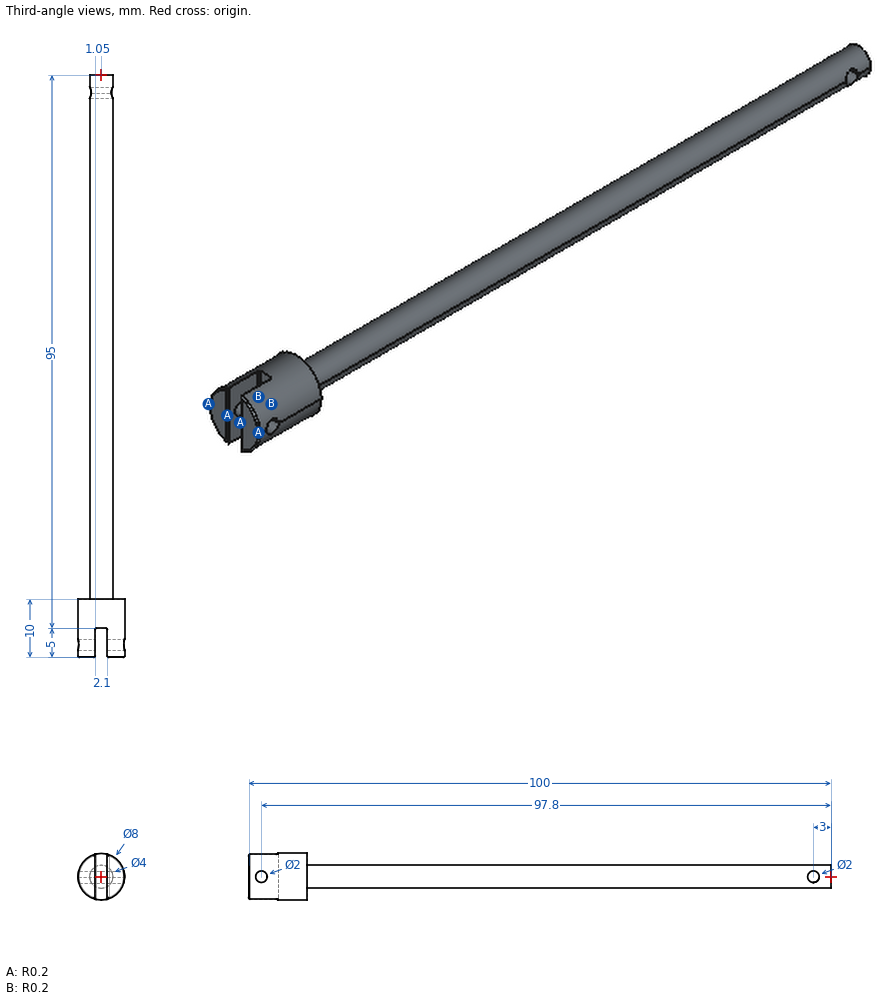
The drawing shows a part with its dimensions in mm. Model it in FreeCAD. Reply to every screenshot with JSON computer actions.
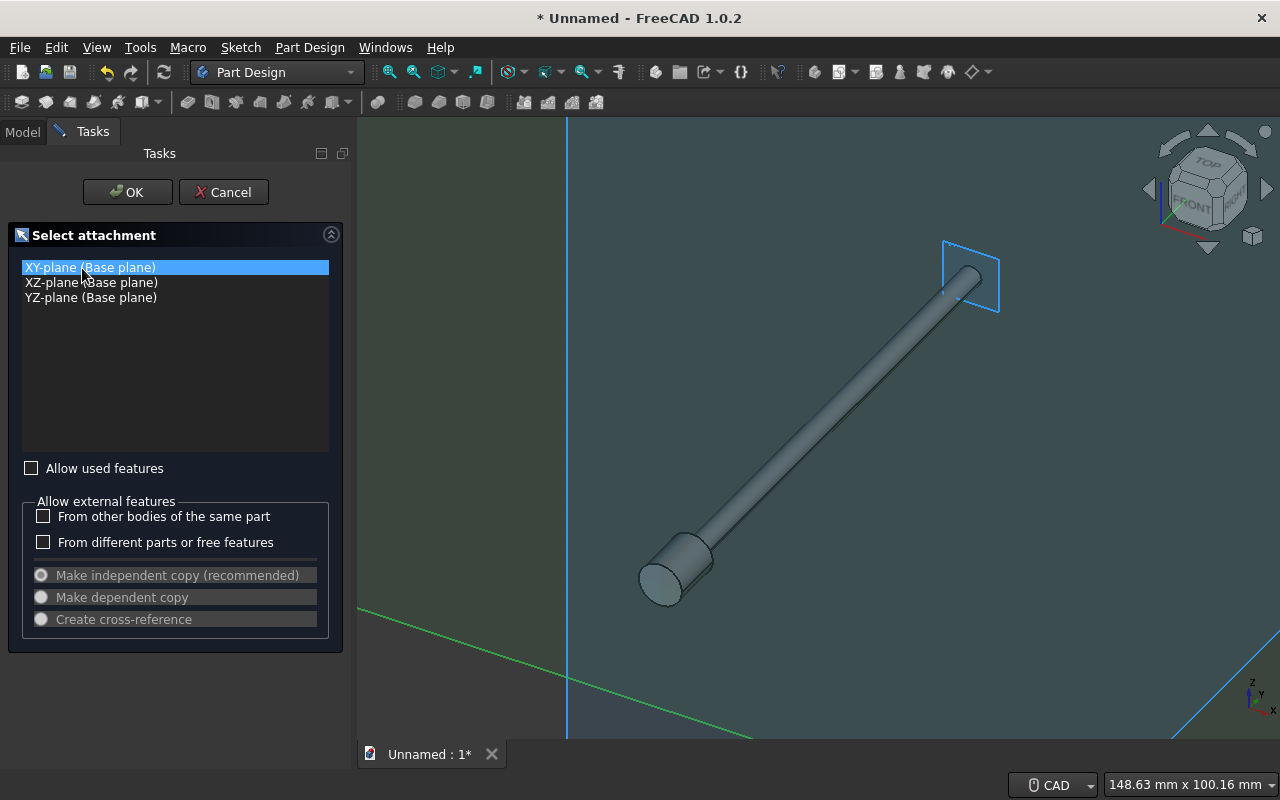
{"action": "left_click", "coordinate": [128, 192]}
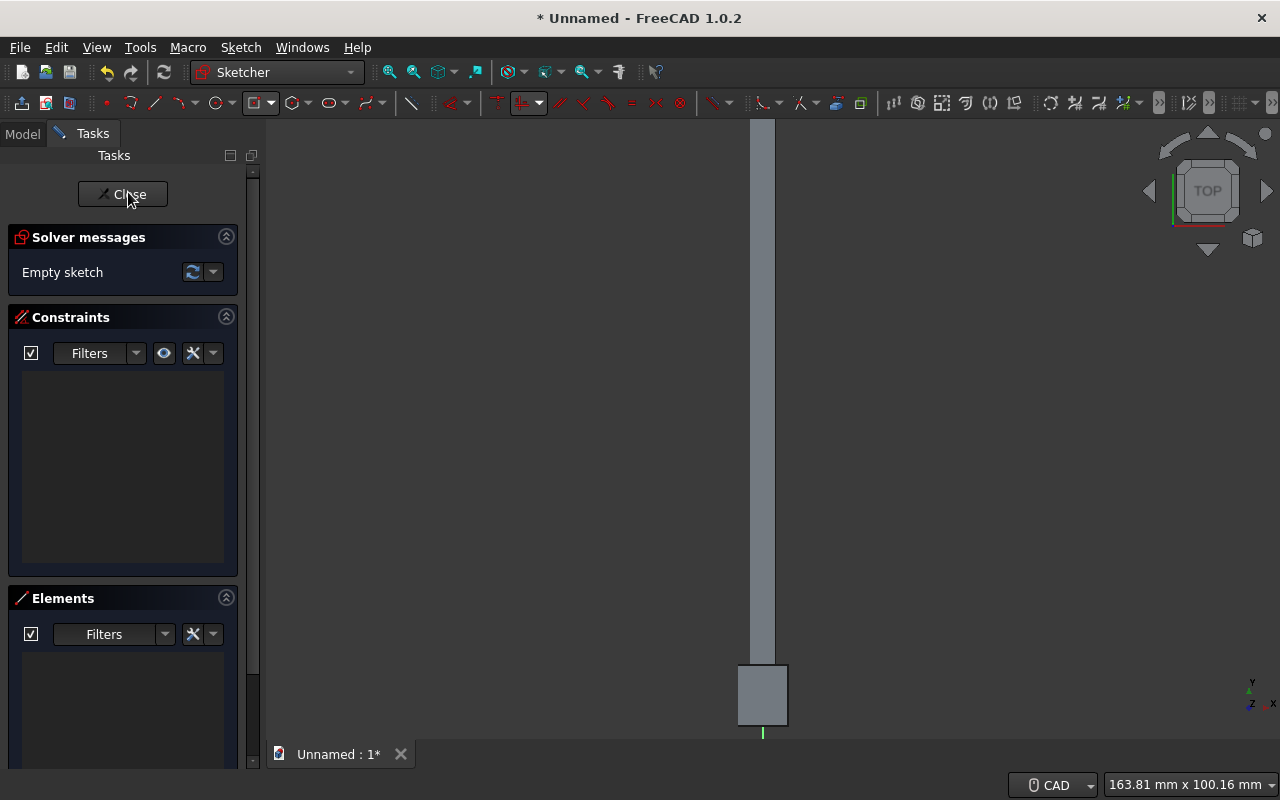
{"action": "key", "text": "q s"}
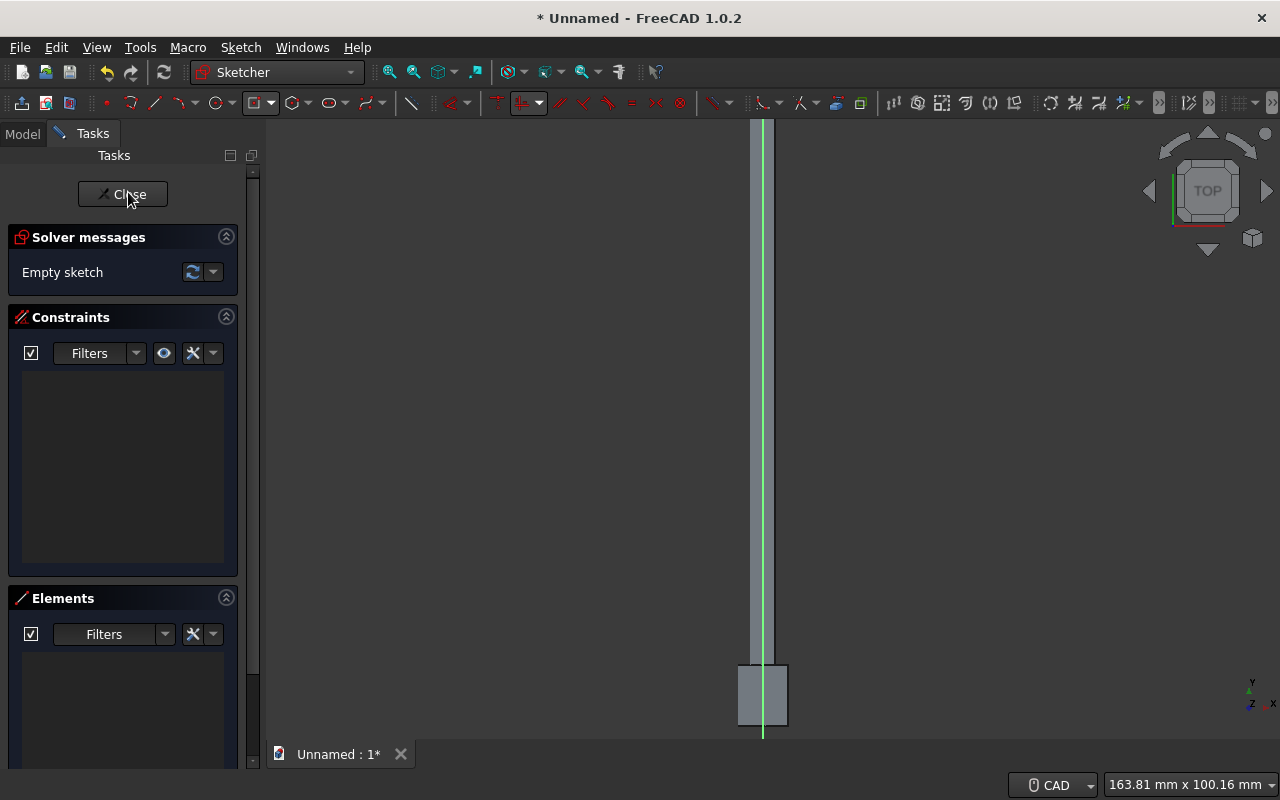
{"action": "scroll", "coordinate": [704, 429], "scroll_direction": "down", "scroll_amount": 5}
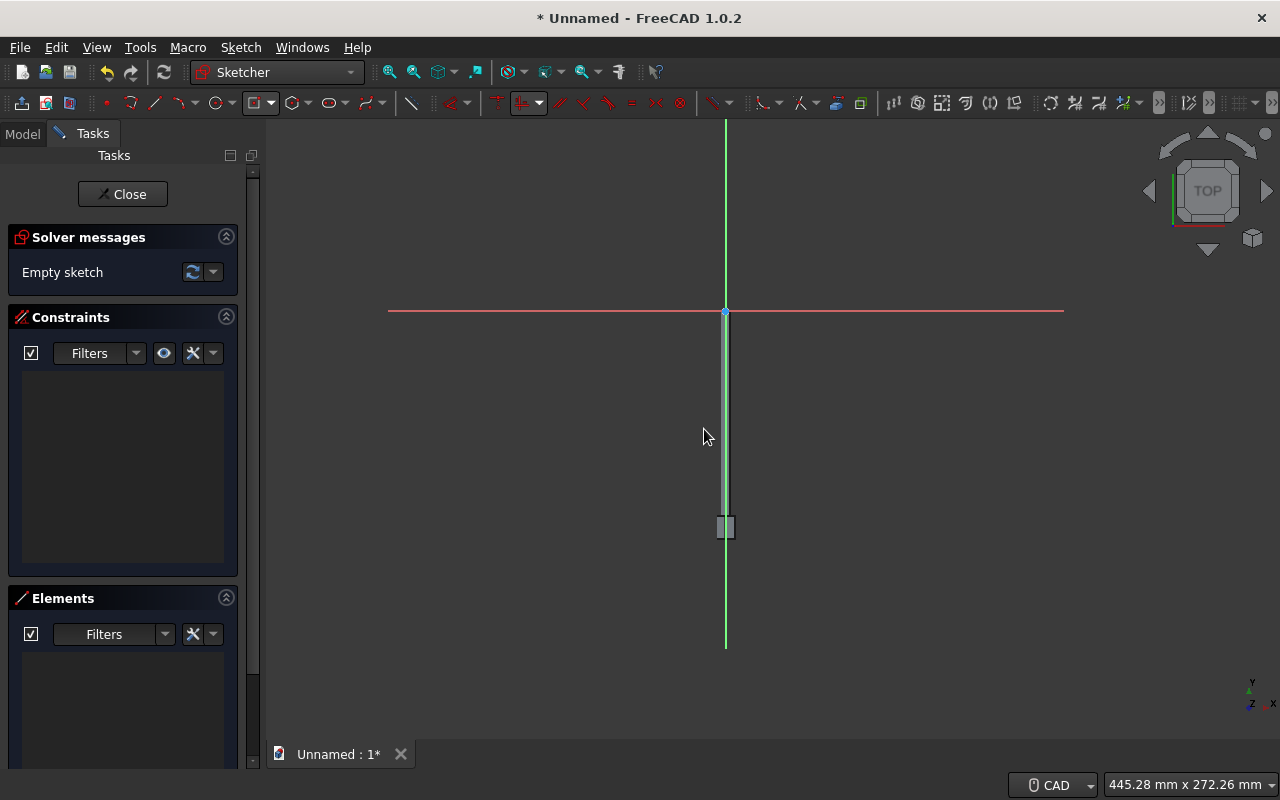
{"action": "scroll", "coordinate": [727, 539], "scroll_direction": "up", "scroll_amount": 15}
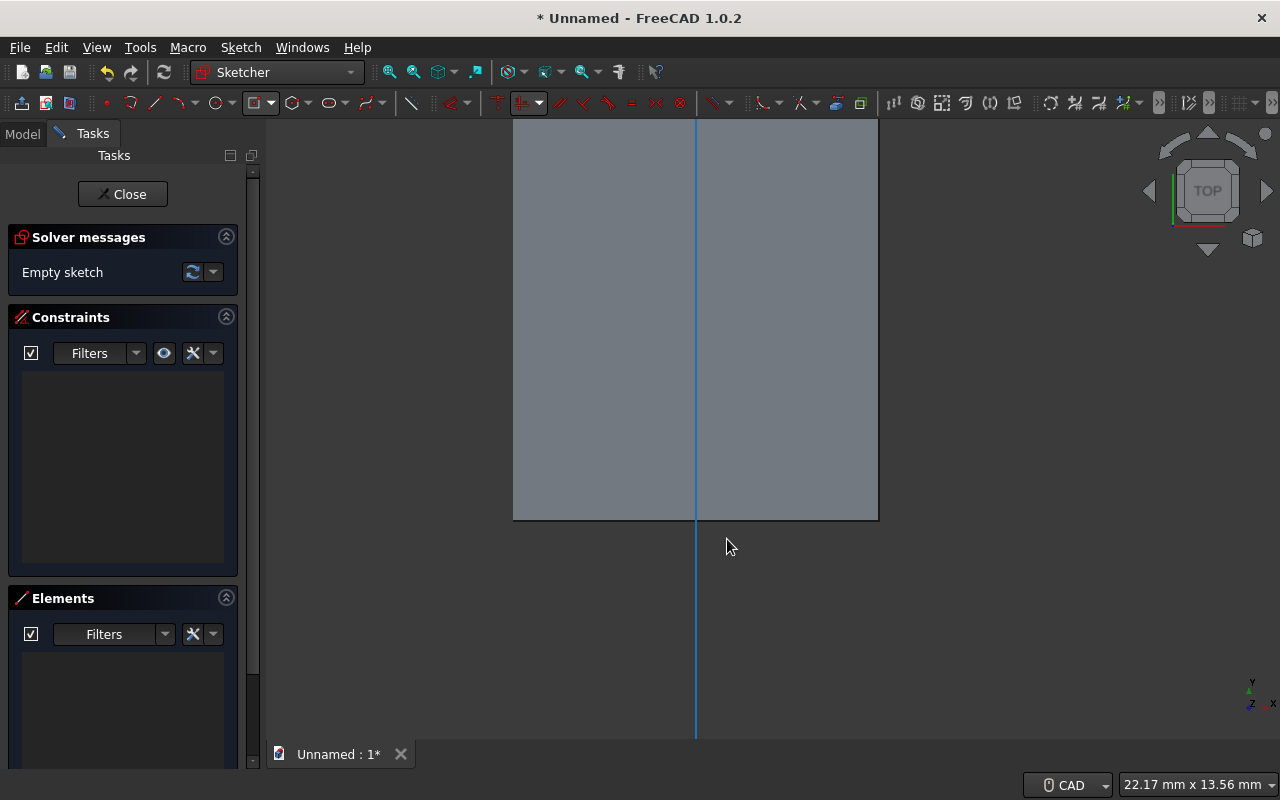
{"action": "scroll", "coordinate": [685, 379], "scroll_direction": "up", "scroll_amount": 3}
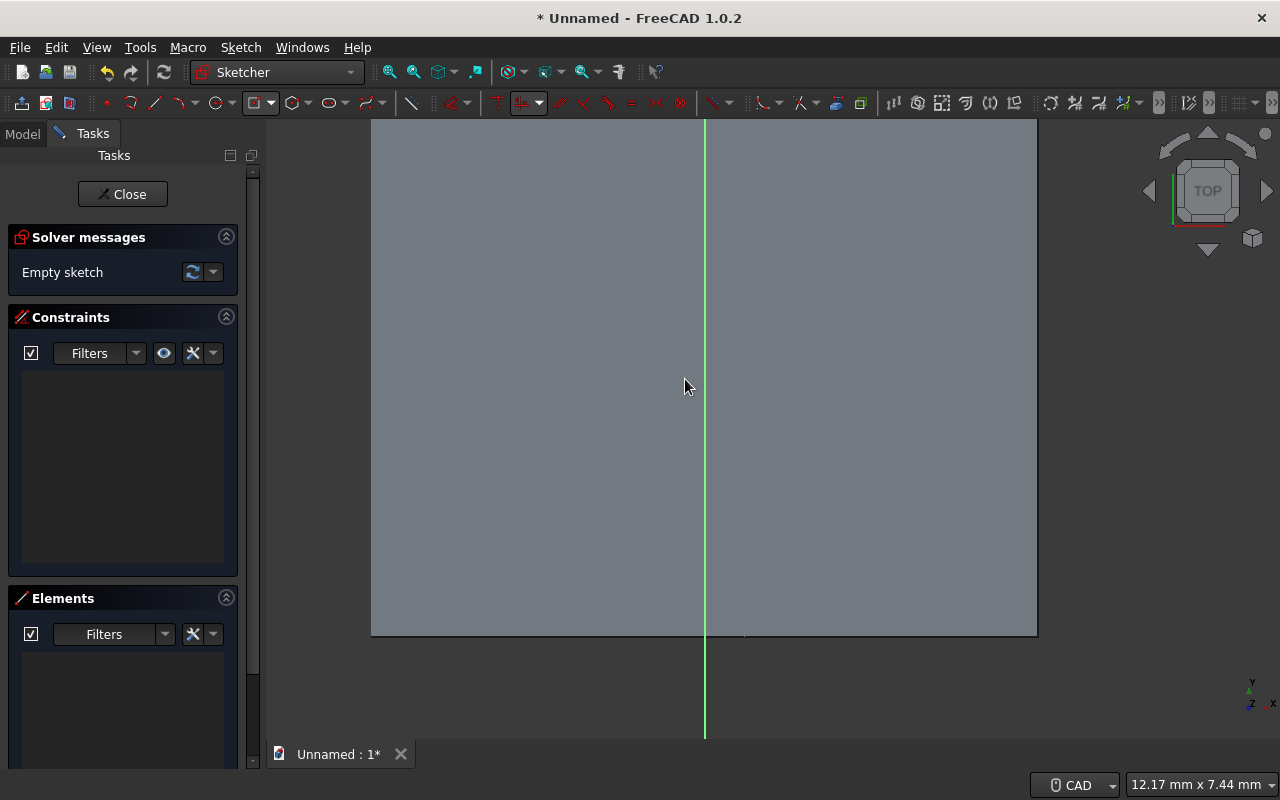
{"action": "key", "text": "g r"}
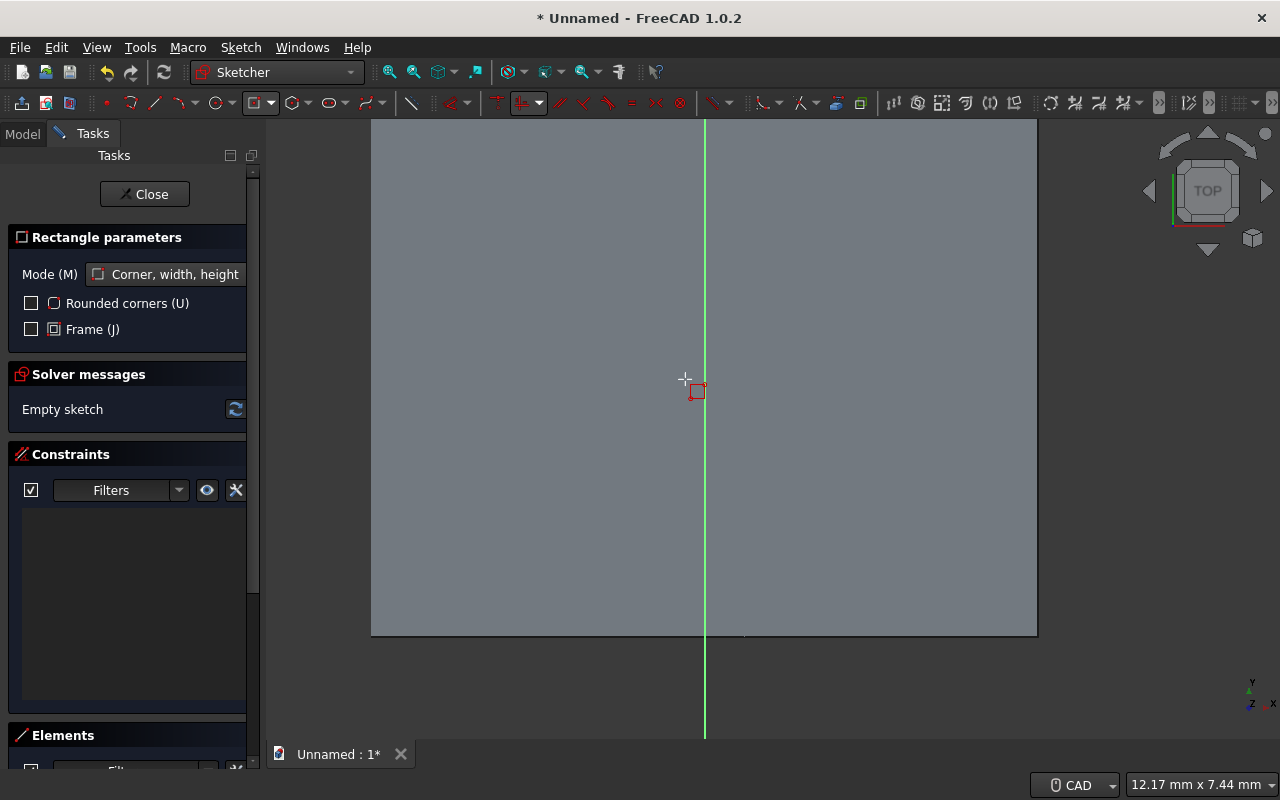
{"action": "left_click", "coordinate": [617, 221]}
{"action": "left_click", "coordinate": [792, 637]}
{"action": "key", "text": "Escape"}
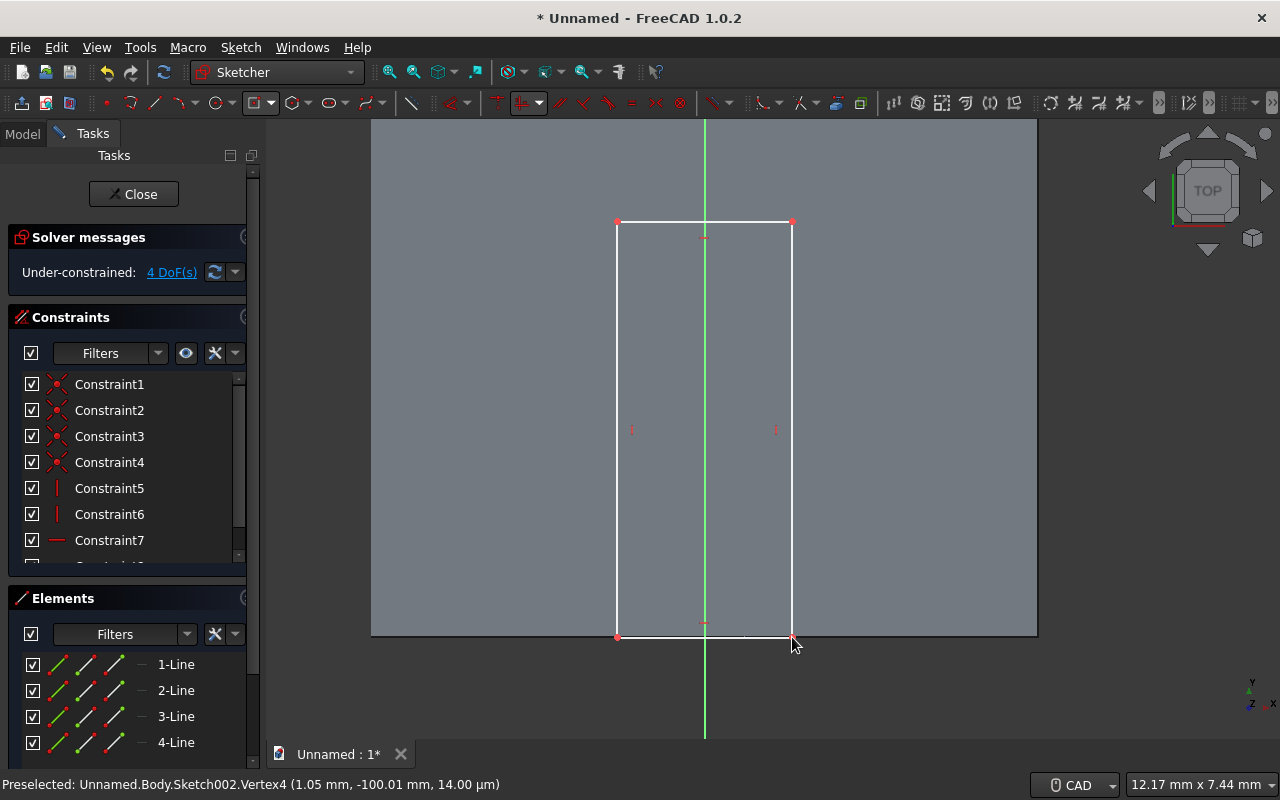
{"action": "left_click", "coordinate": [450, 104]}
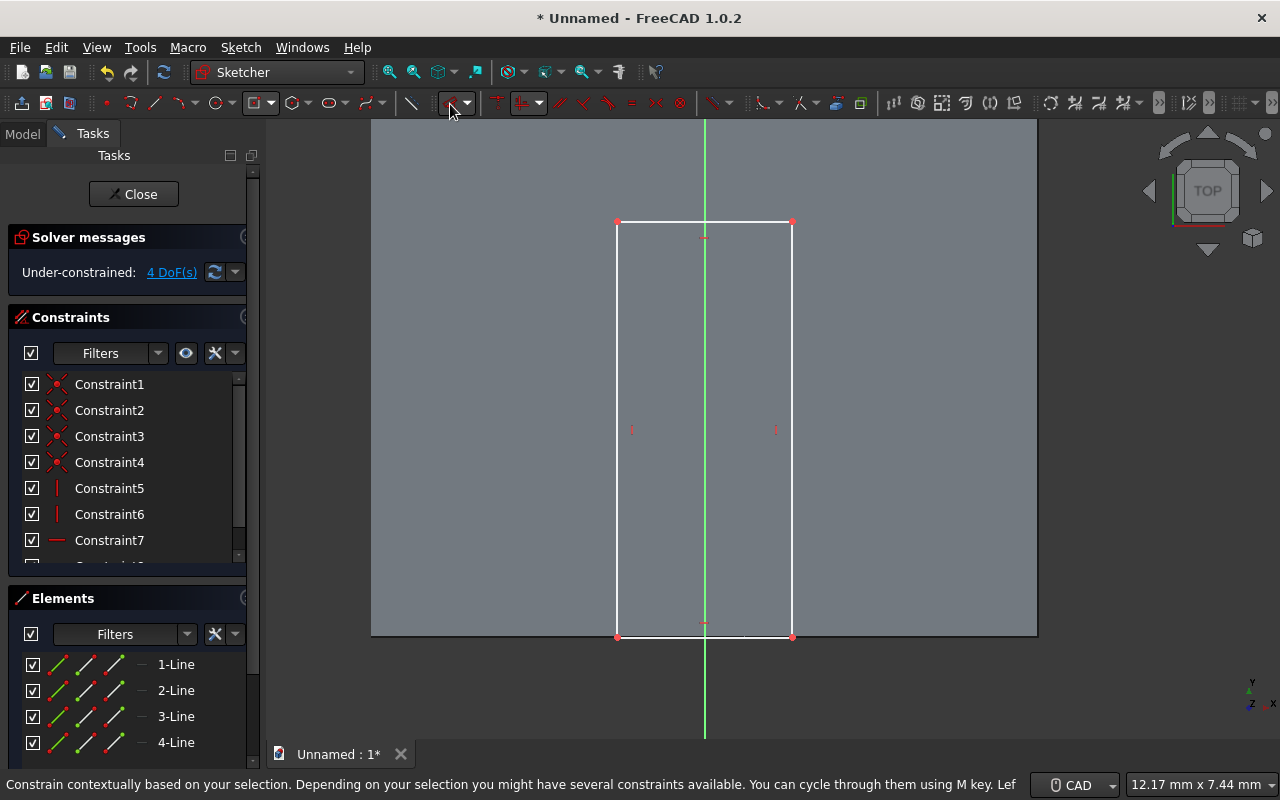
{"action": "left_click", "coordinate": [617, 347]}
{"action": "left_click", "coordinate": [583, 430]}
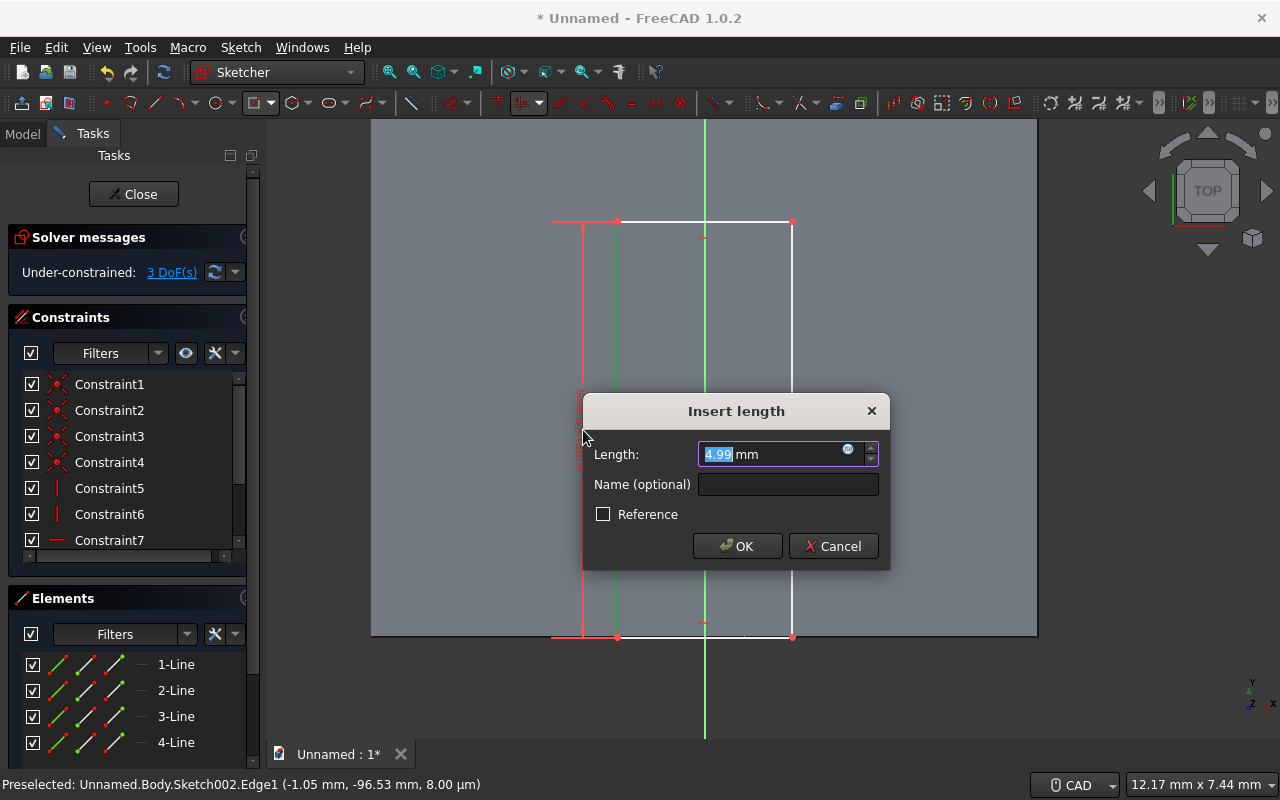
{"action": "type", "text": "5"}
{"action": "key", "text": "Return"}